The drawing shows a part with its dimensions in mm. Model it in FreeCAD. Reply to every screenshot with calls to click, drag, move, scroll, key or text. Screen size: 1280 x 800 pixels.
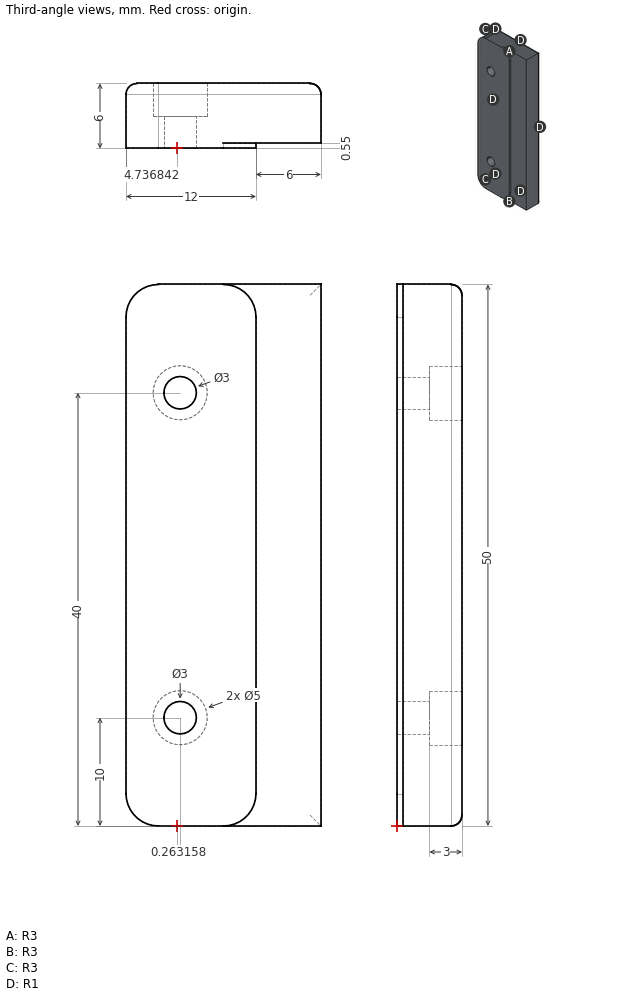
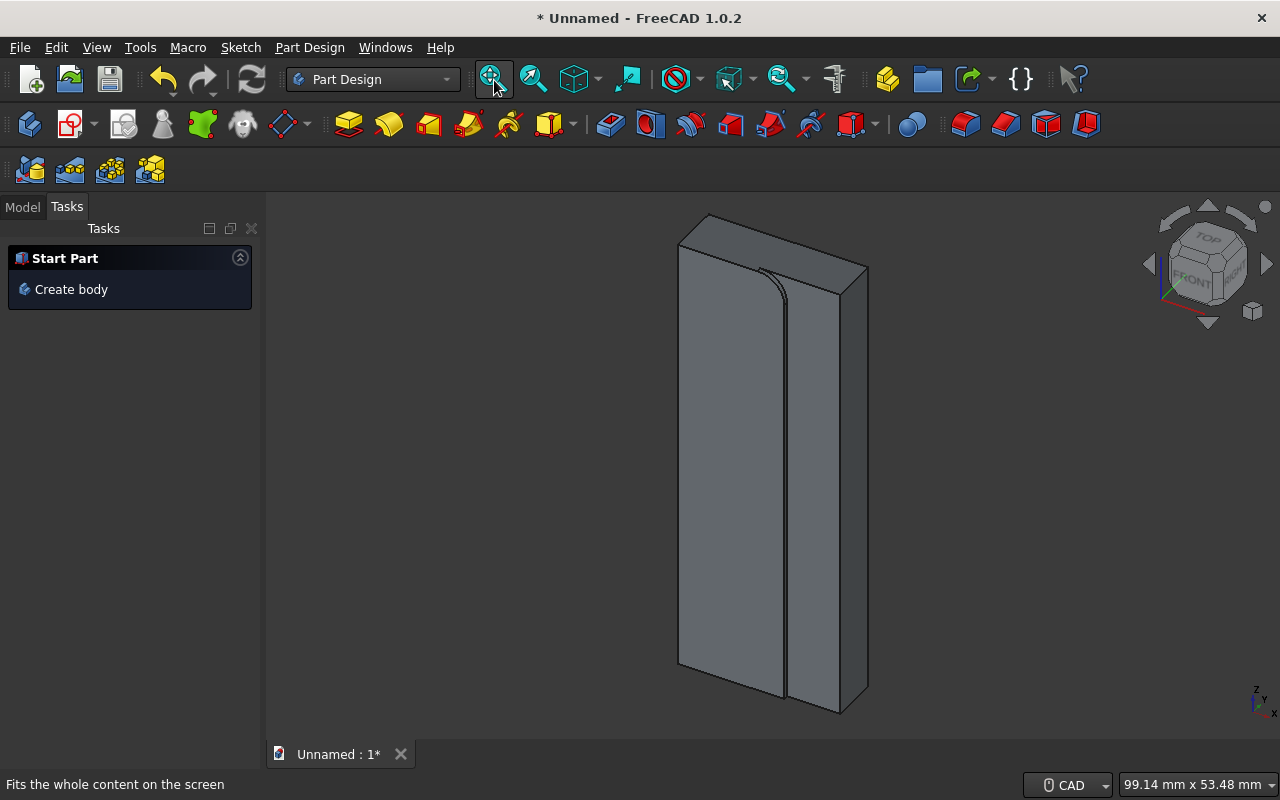
key(4)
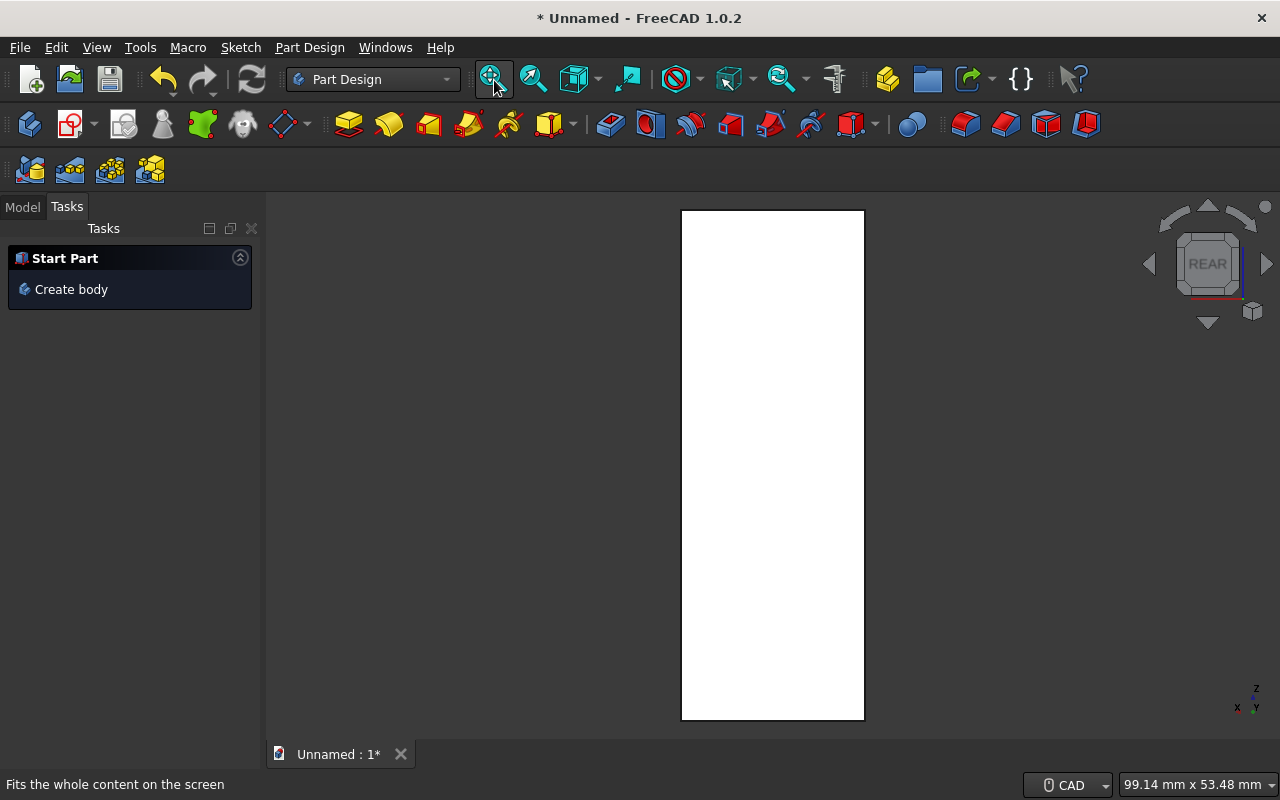
click(773, 318)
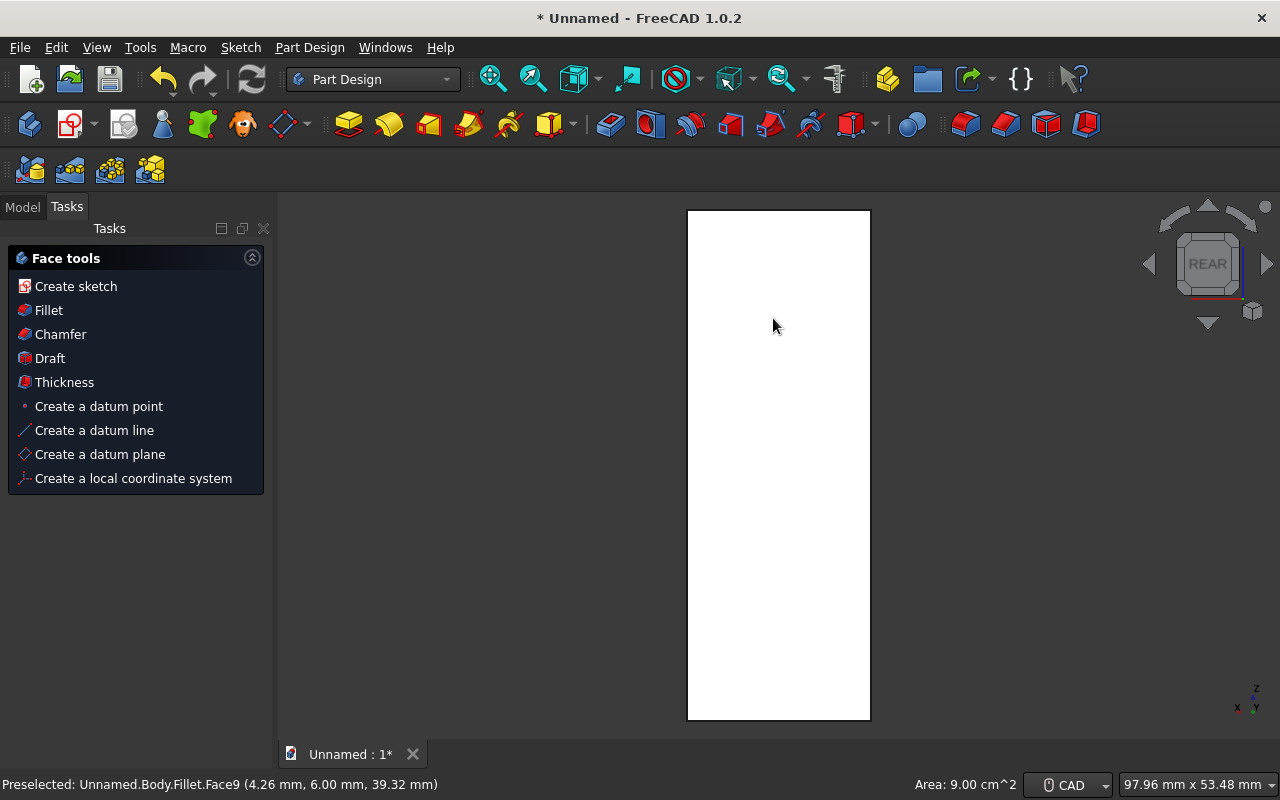
click(70, 124)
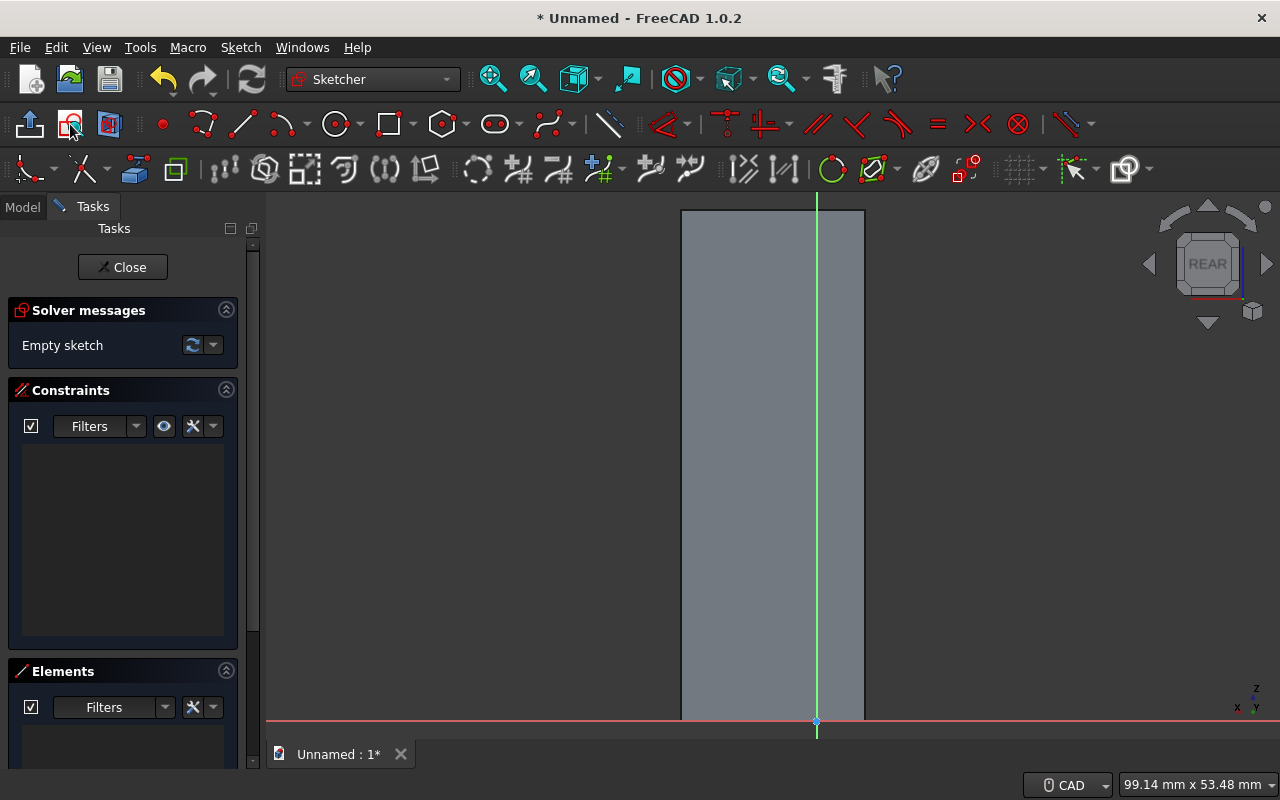
scroll(294, 292, down, 1)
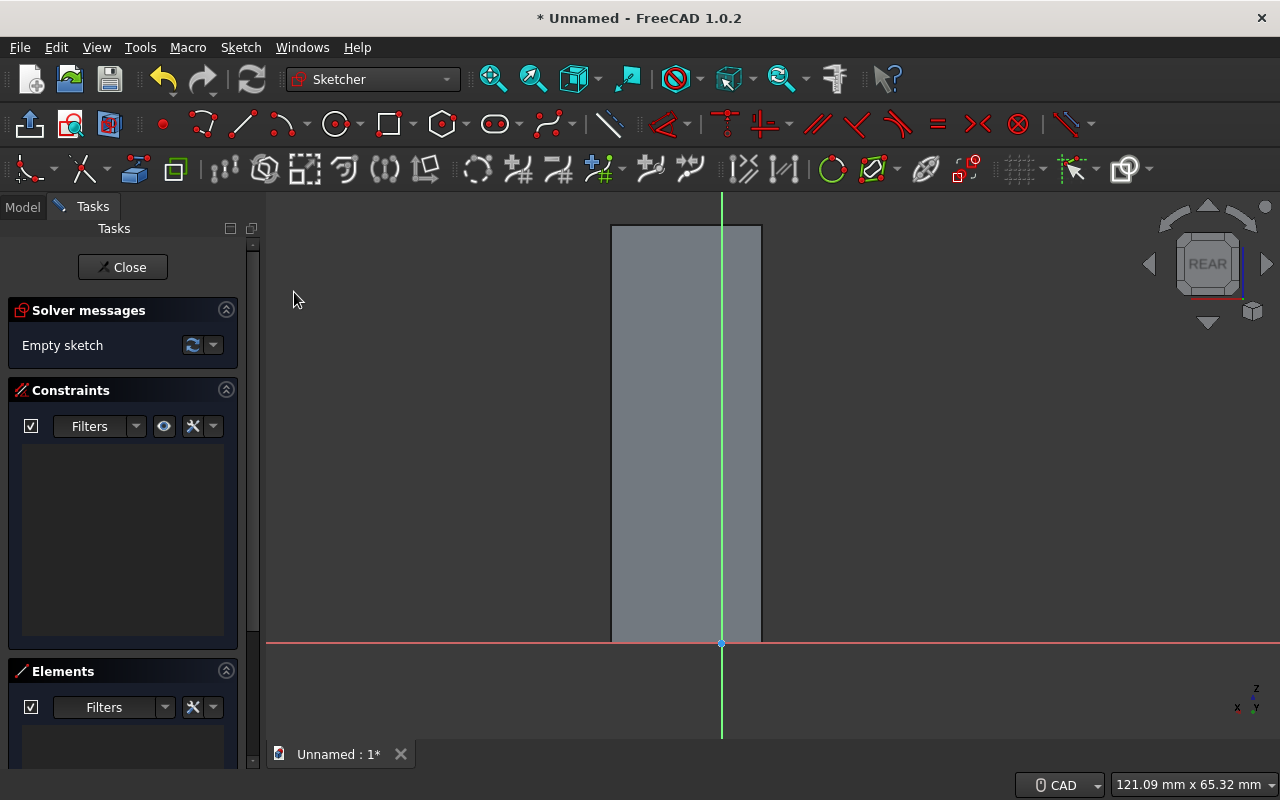
click(336, 124)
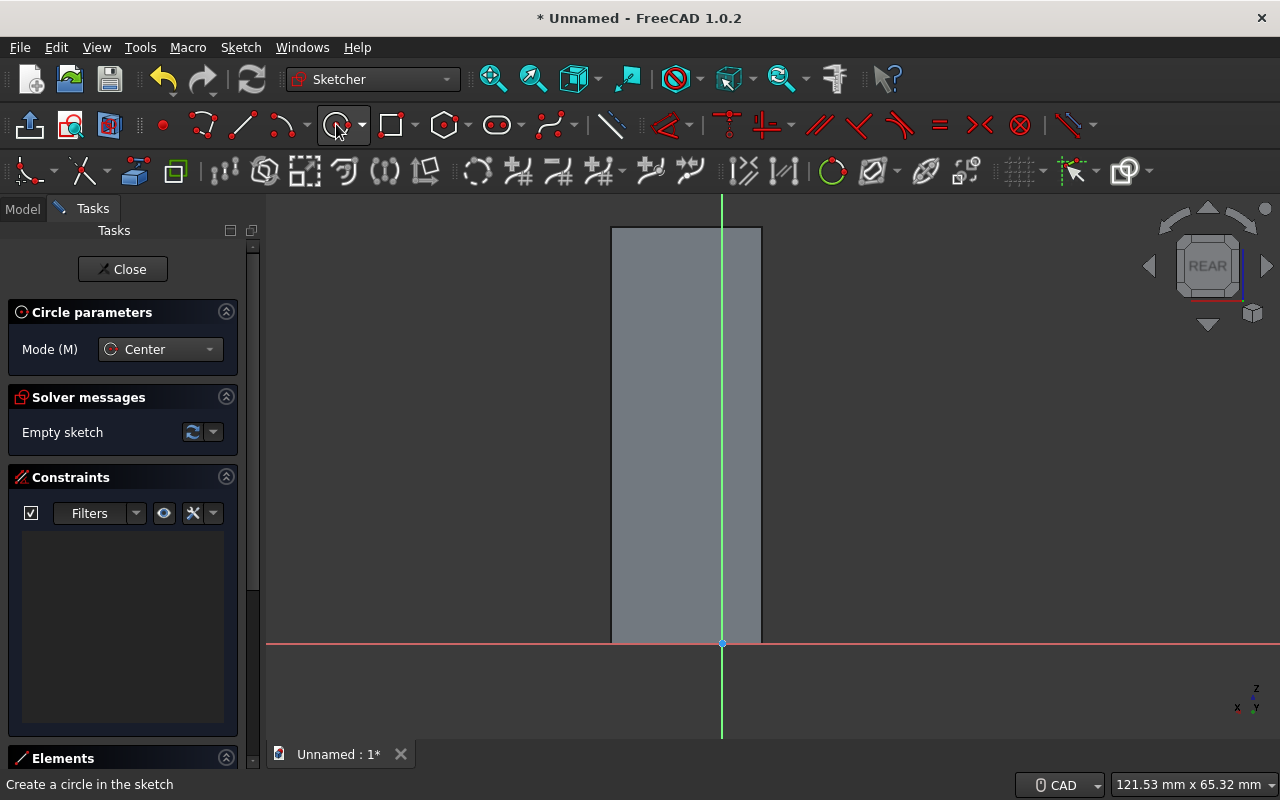
scroll(720, 560, up, 10)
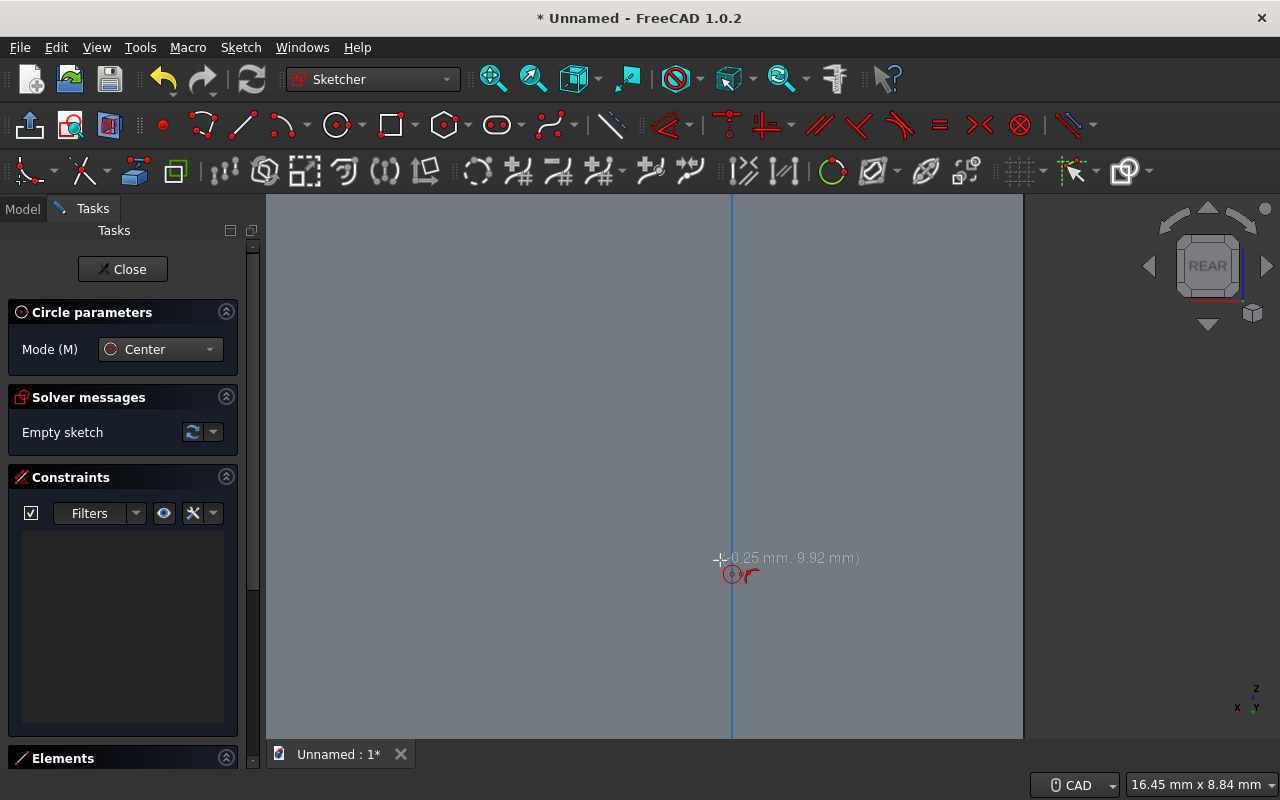
click(716, 558)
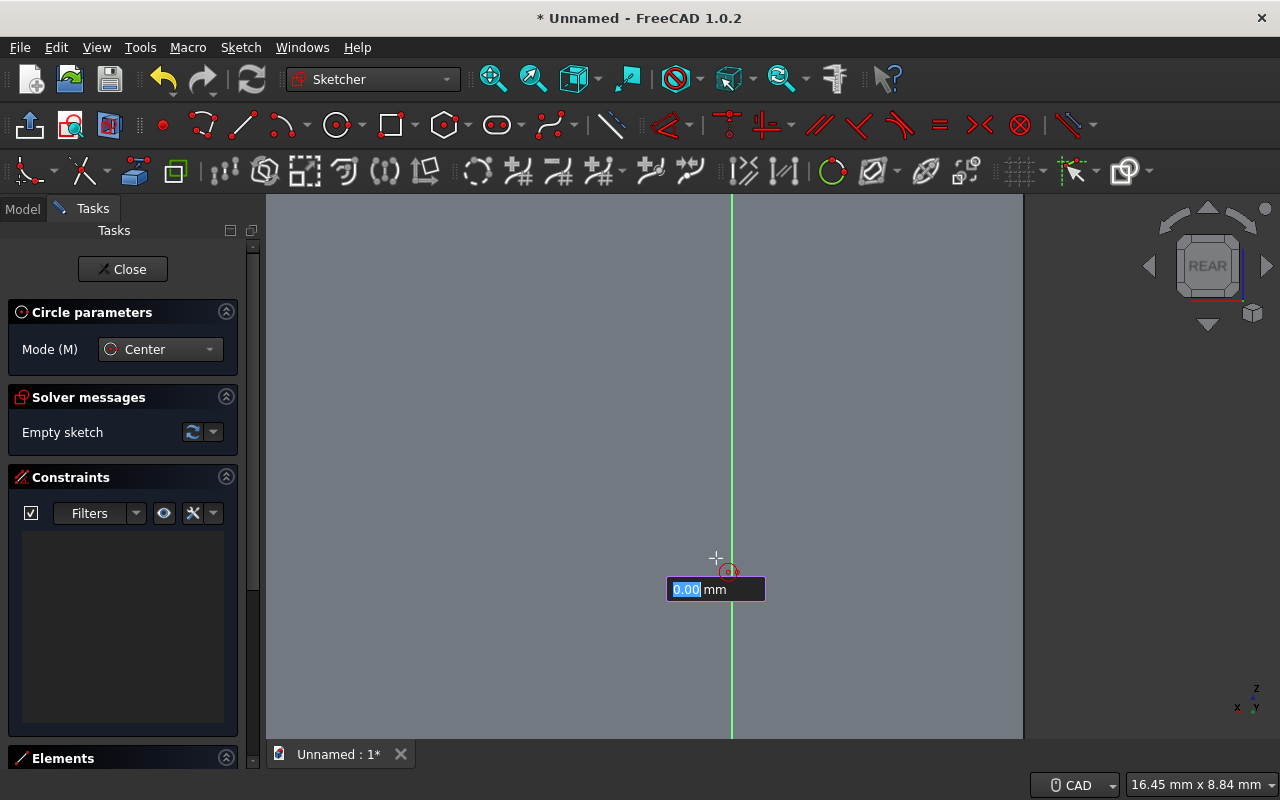
scroll(703, 561, down, 10)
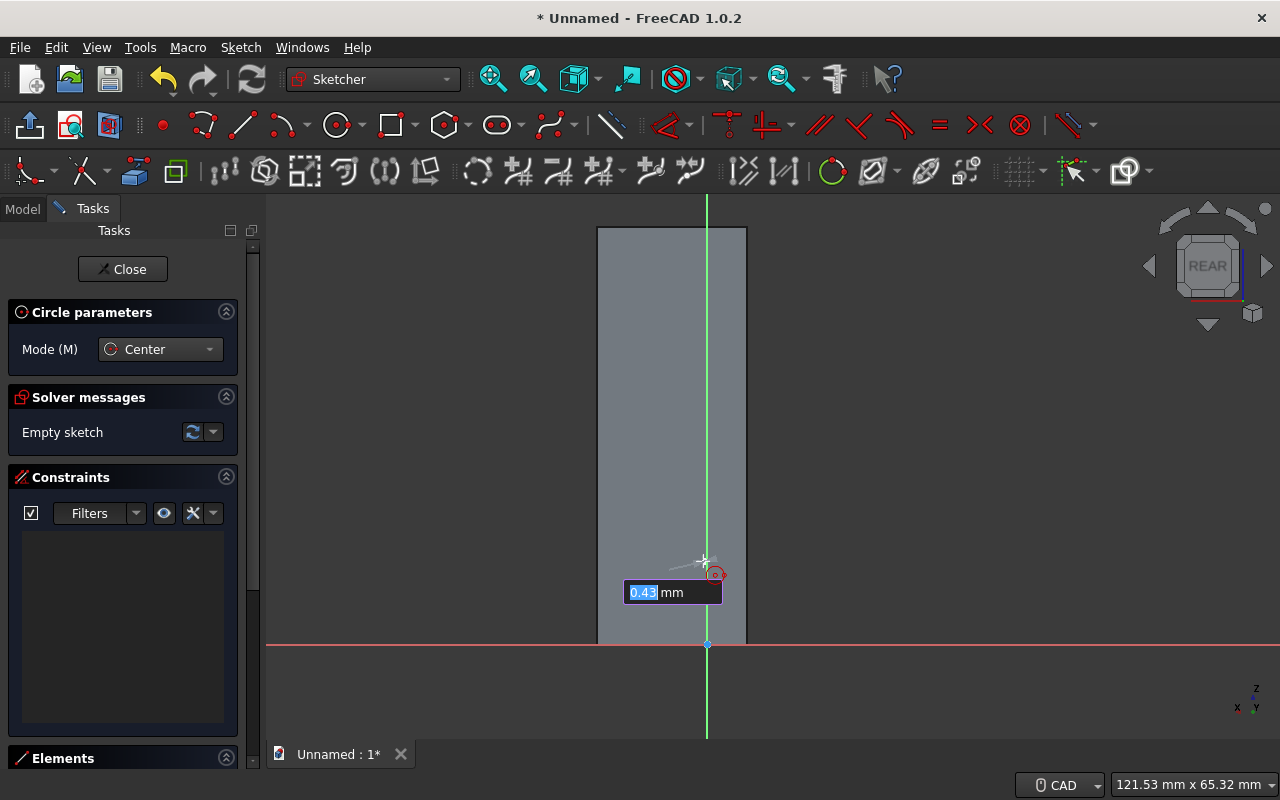
scroll(720, 546, up, 2)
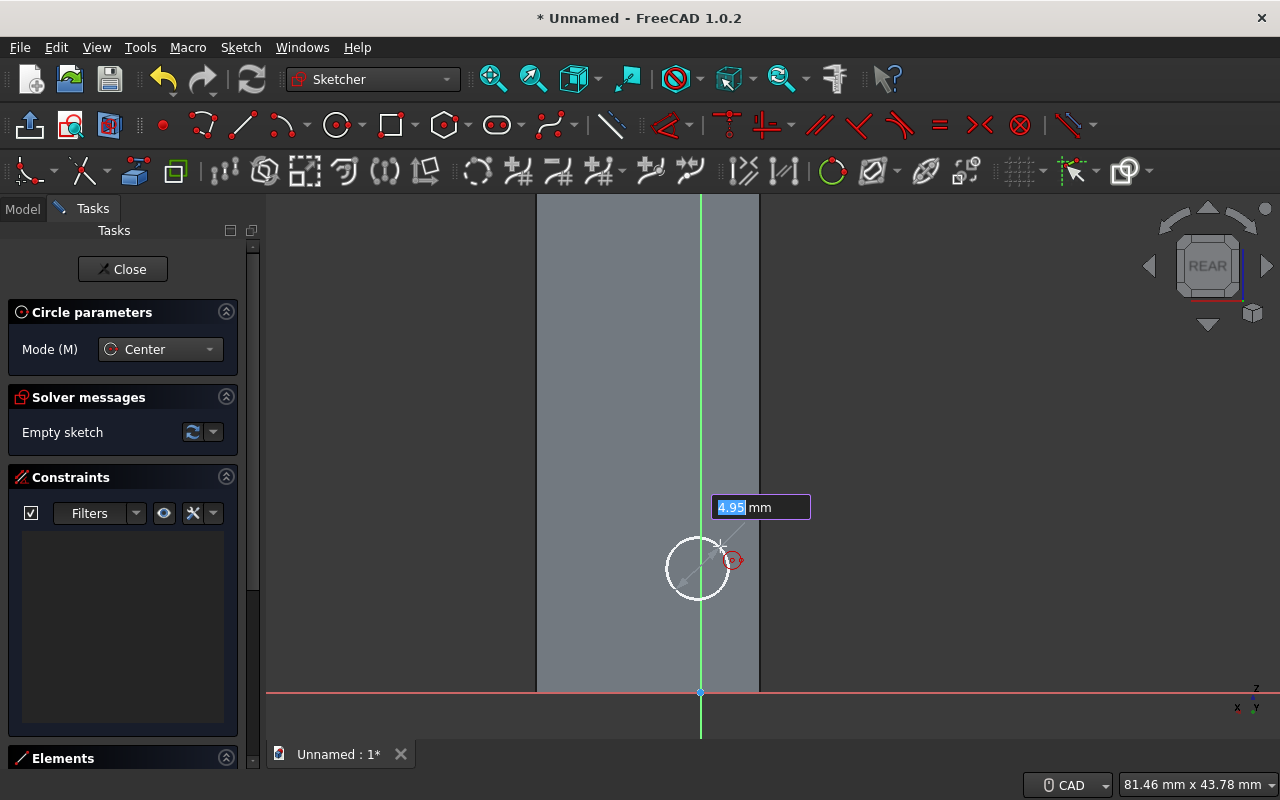
click(720, 546)